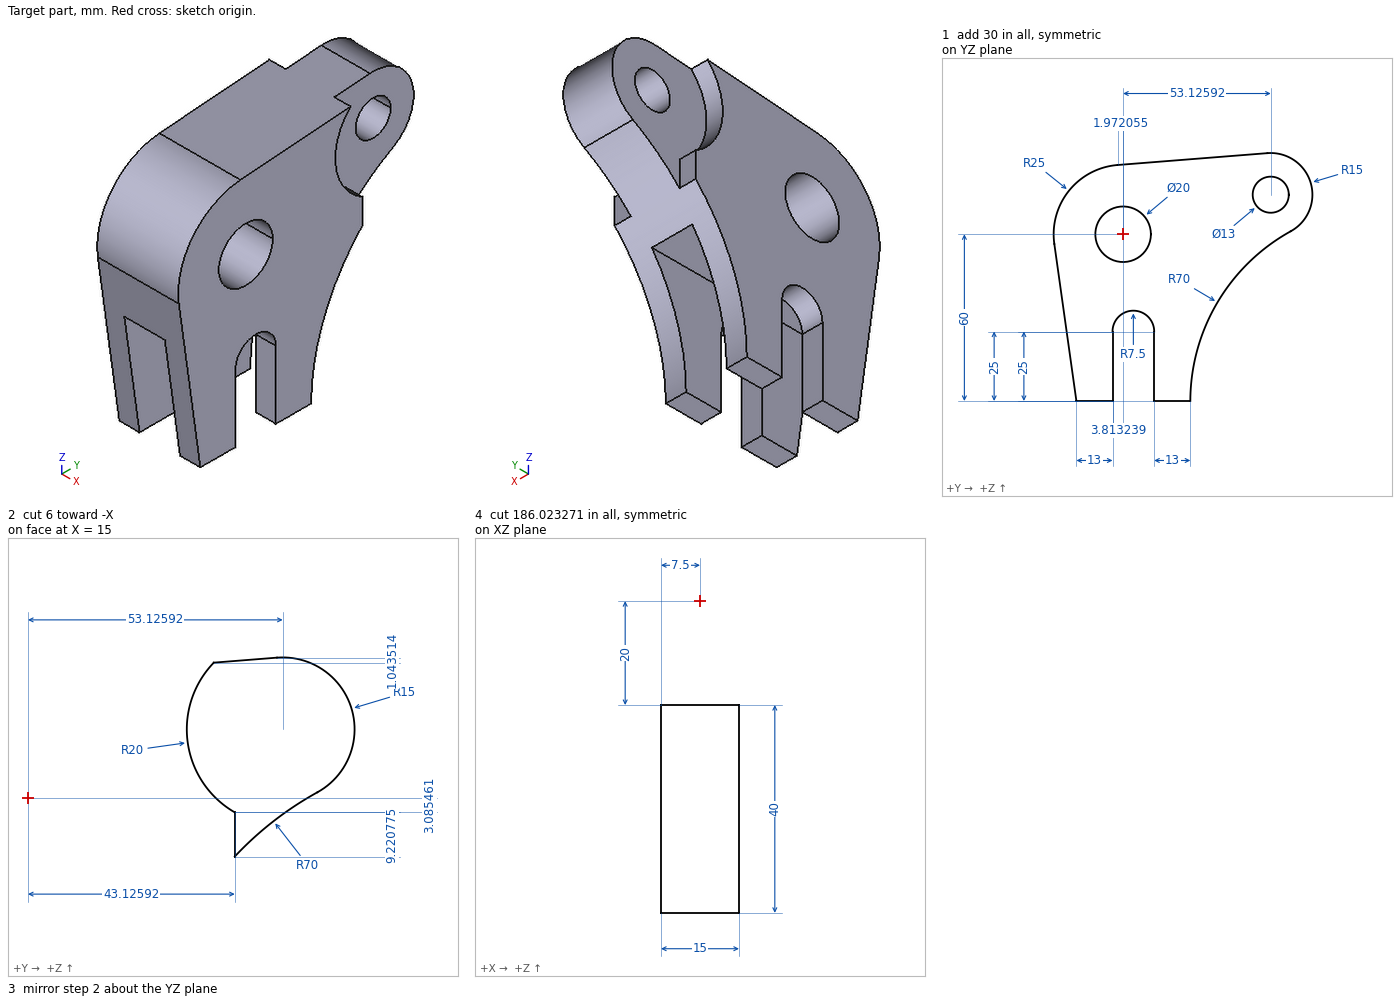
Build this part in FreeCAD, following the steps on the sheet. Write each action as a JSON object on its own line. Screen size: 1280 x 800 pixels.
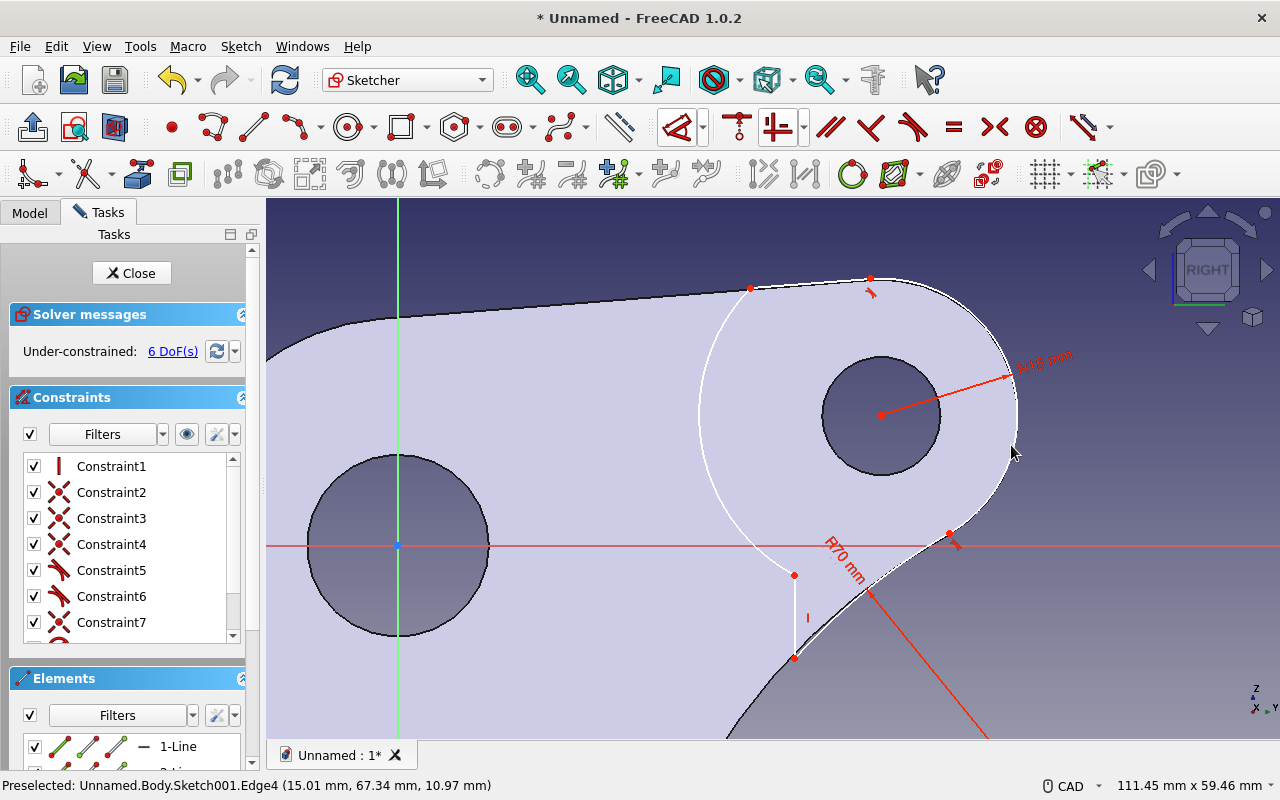
{"action": "left_click", "coordinate": [703, 376]}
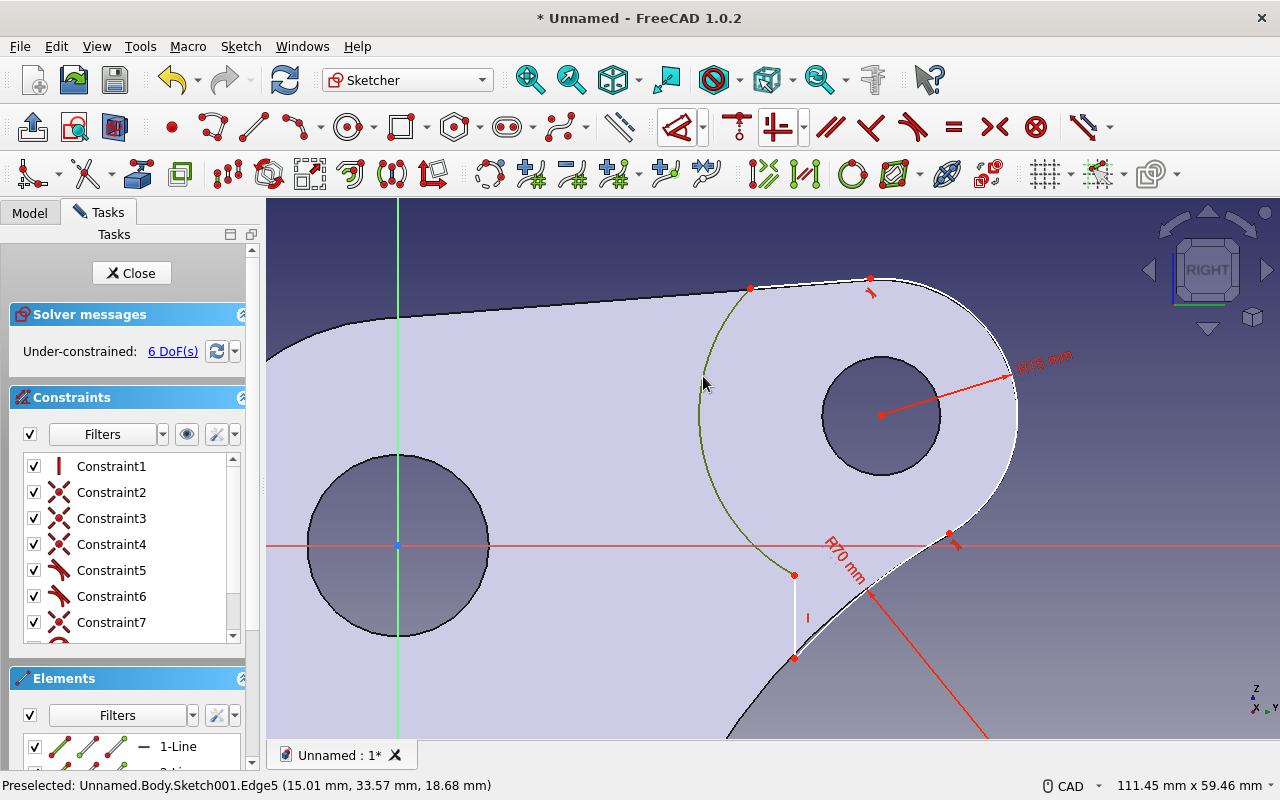
{"action": "left_click", "coordinate": [702, 128]}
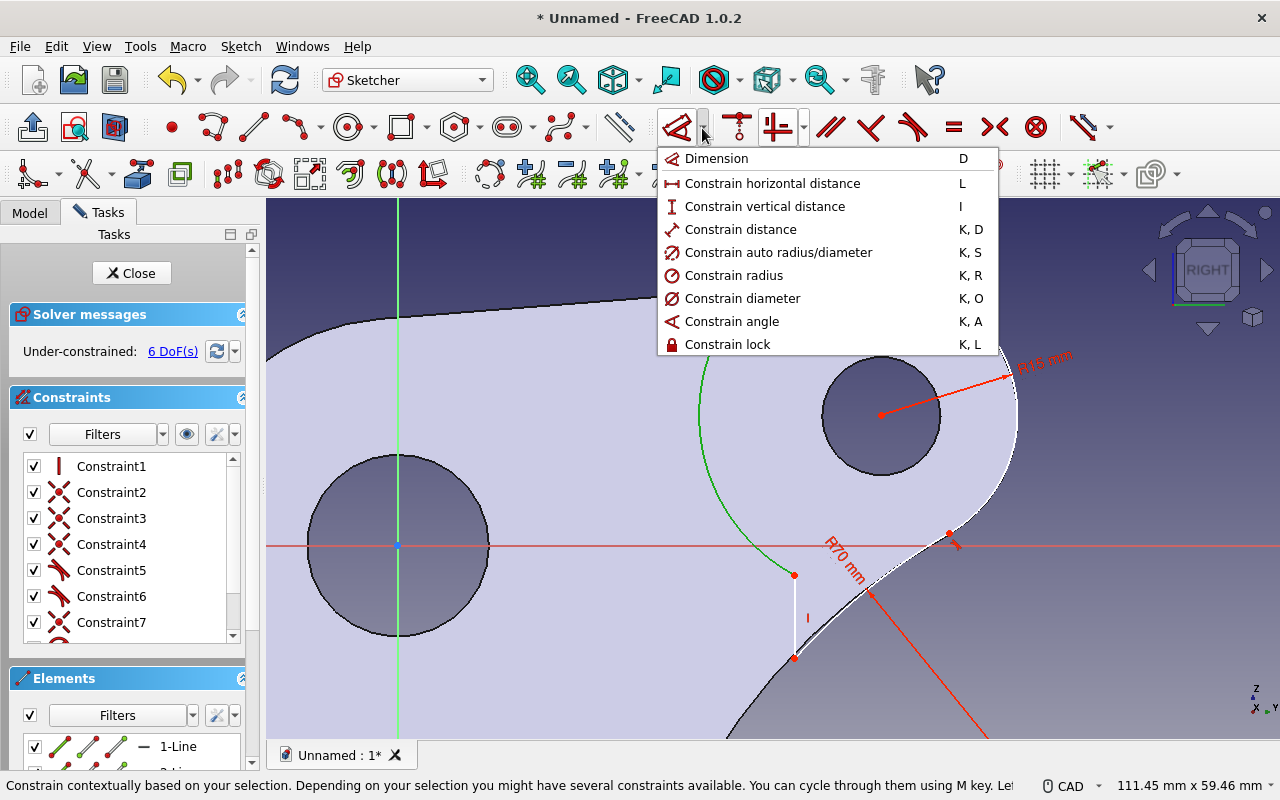
{"action": "left_click", "coordinate": [828, 276]}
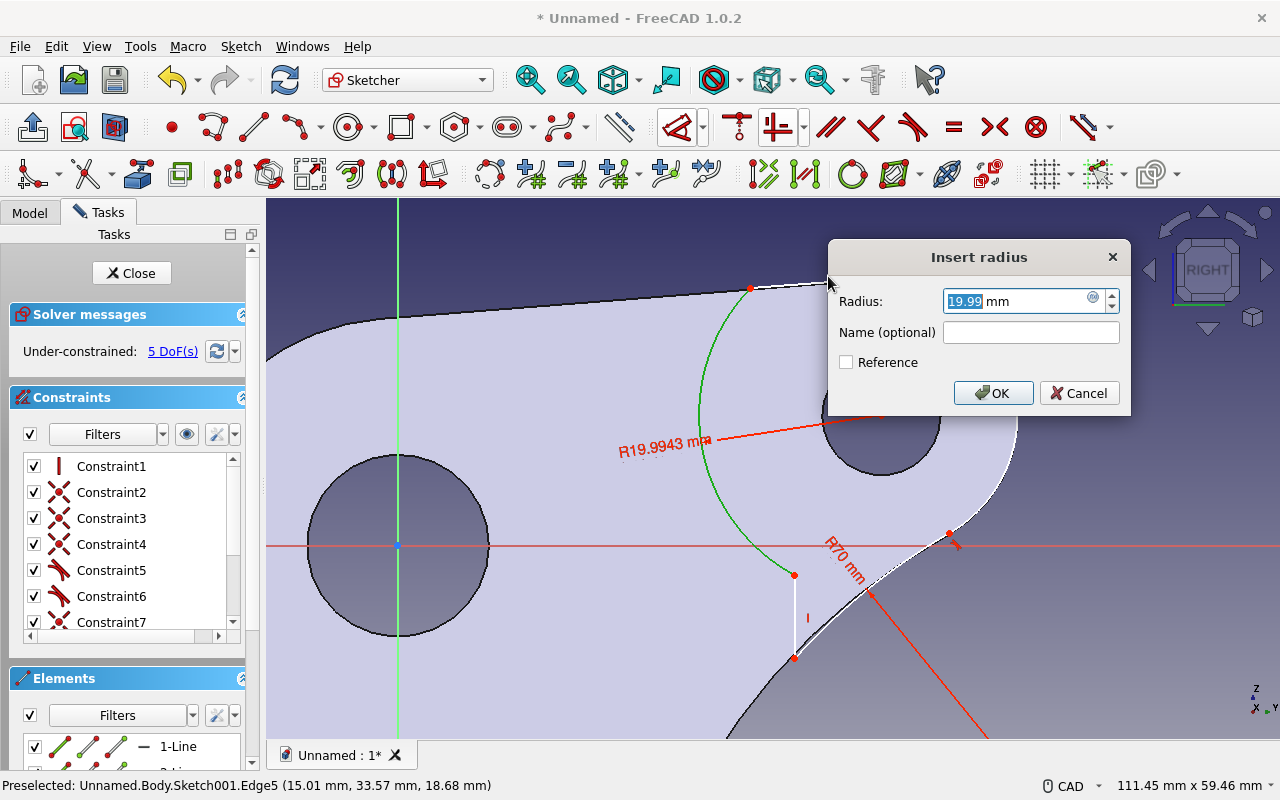
{"action": "type", "text": "20"}
{"action": "key", "text": "Return"}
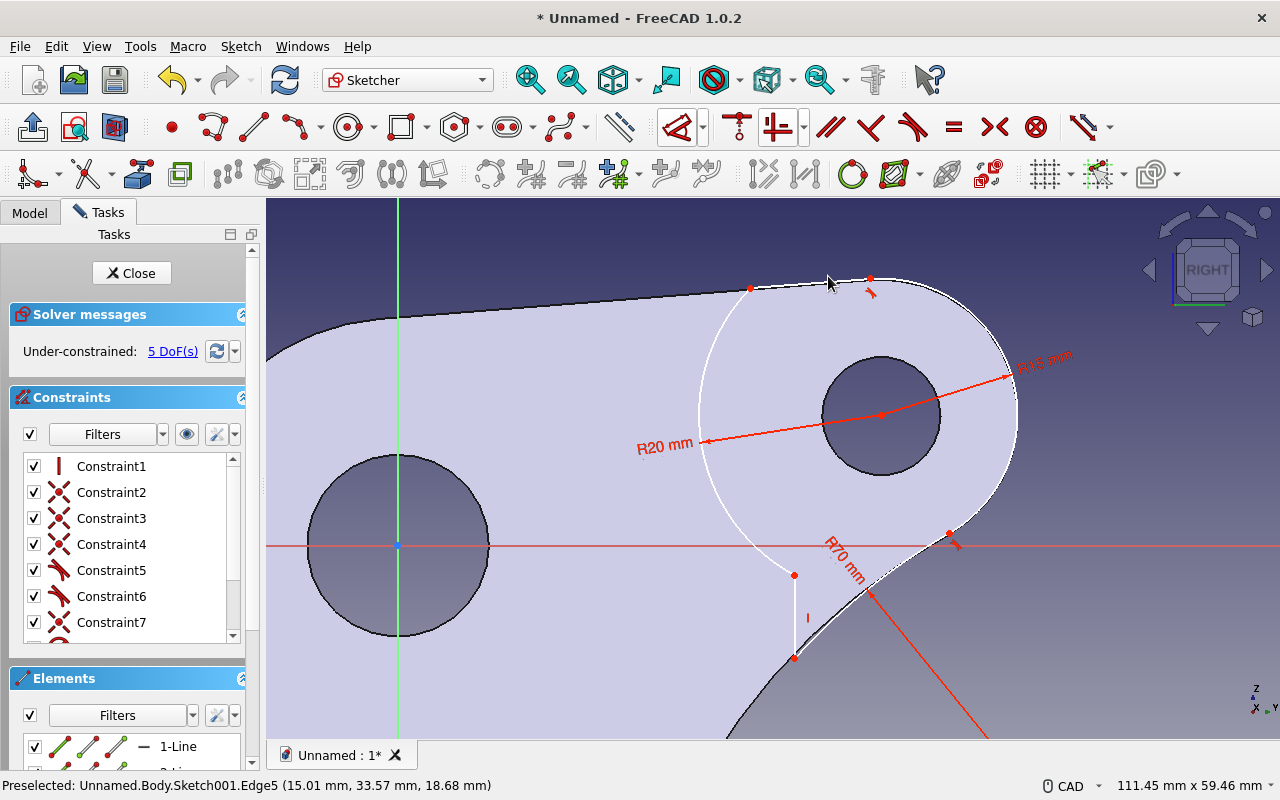
{"action": "left_click", "coordinate": [795, 600]}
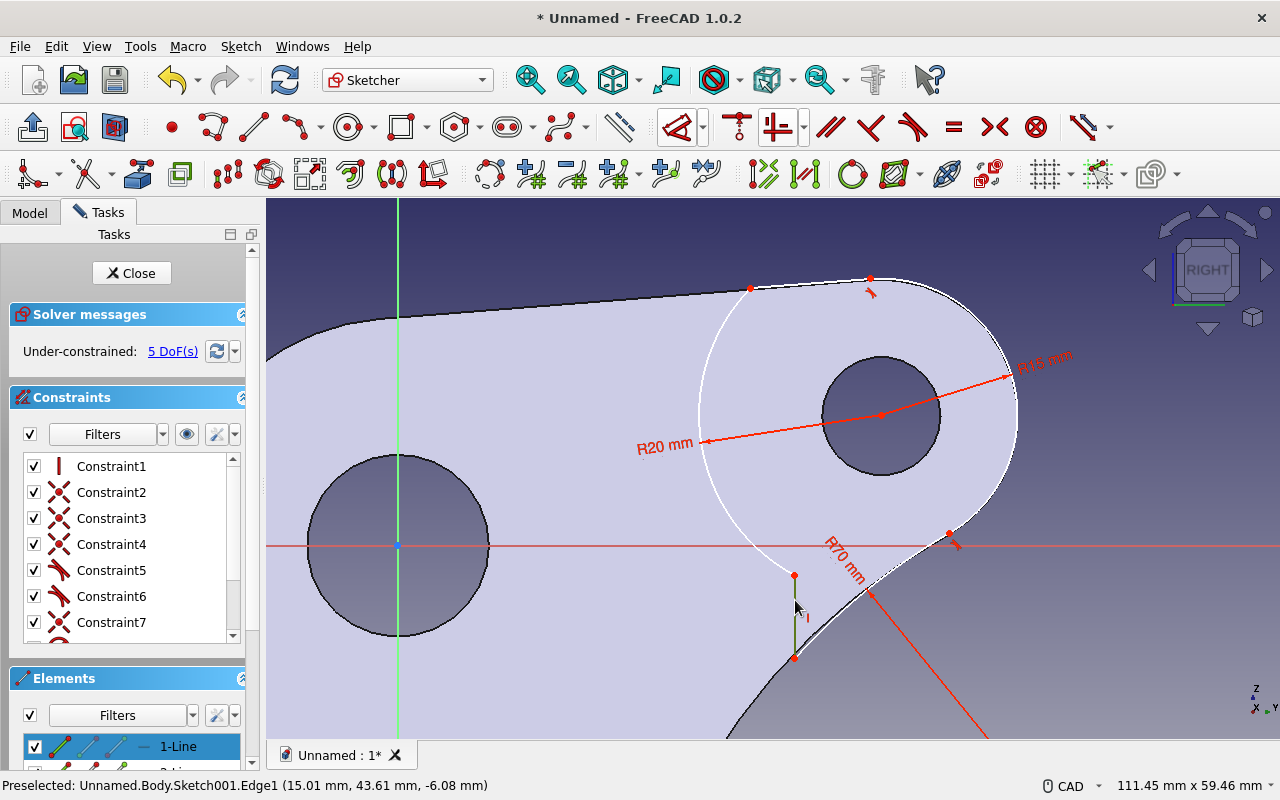
{"action": "left_click", "coordinate": [702, 128]}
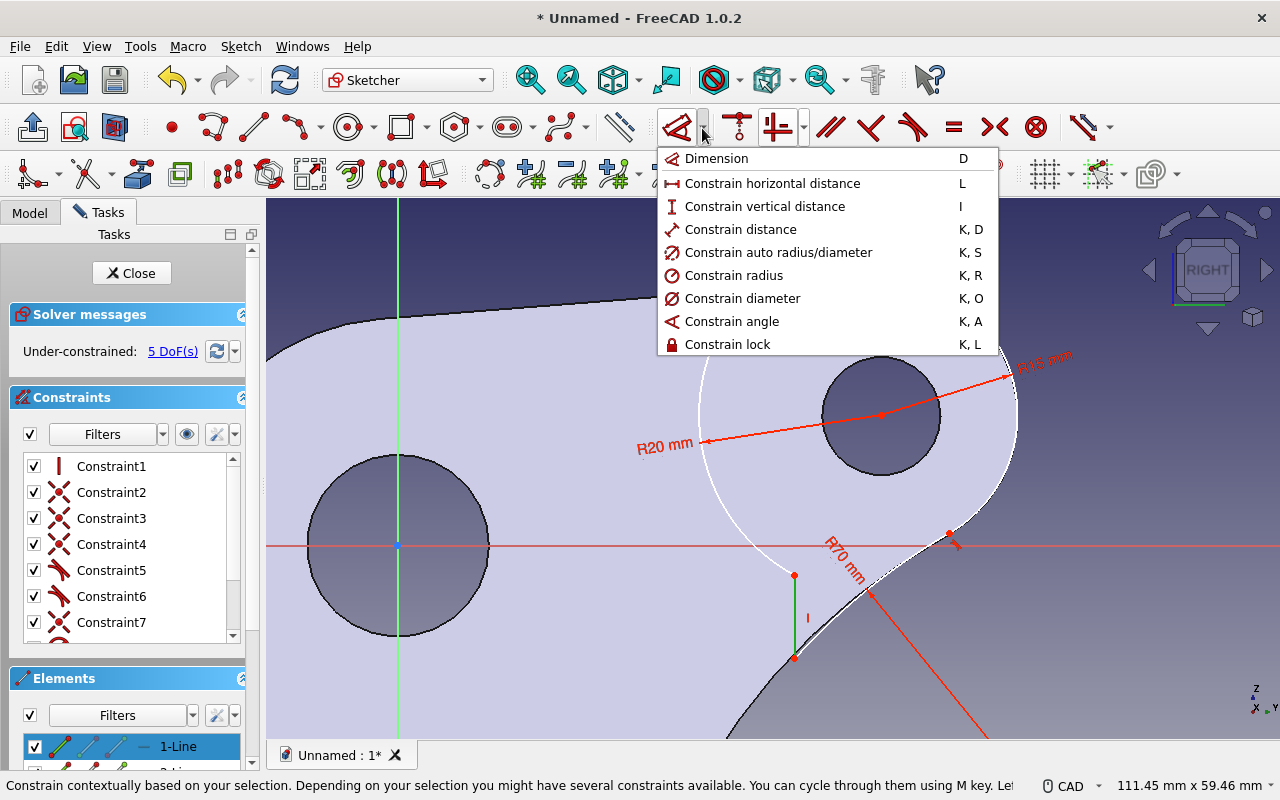
{"action": "left_click", "coordinate": [828, 206]}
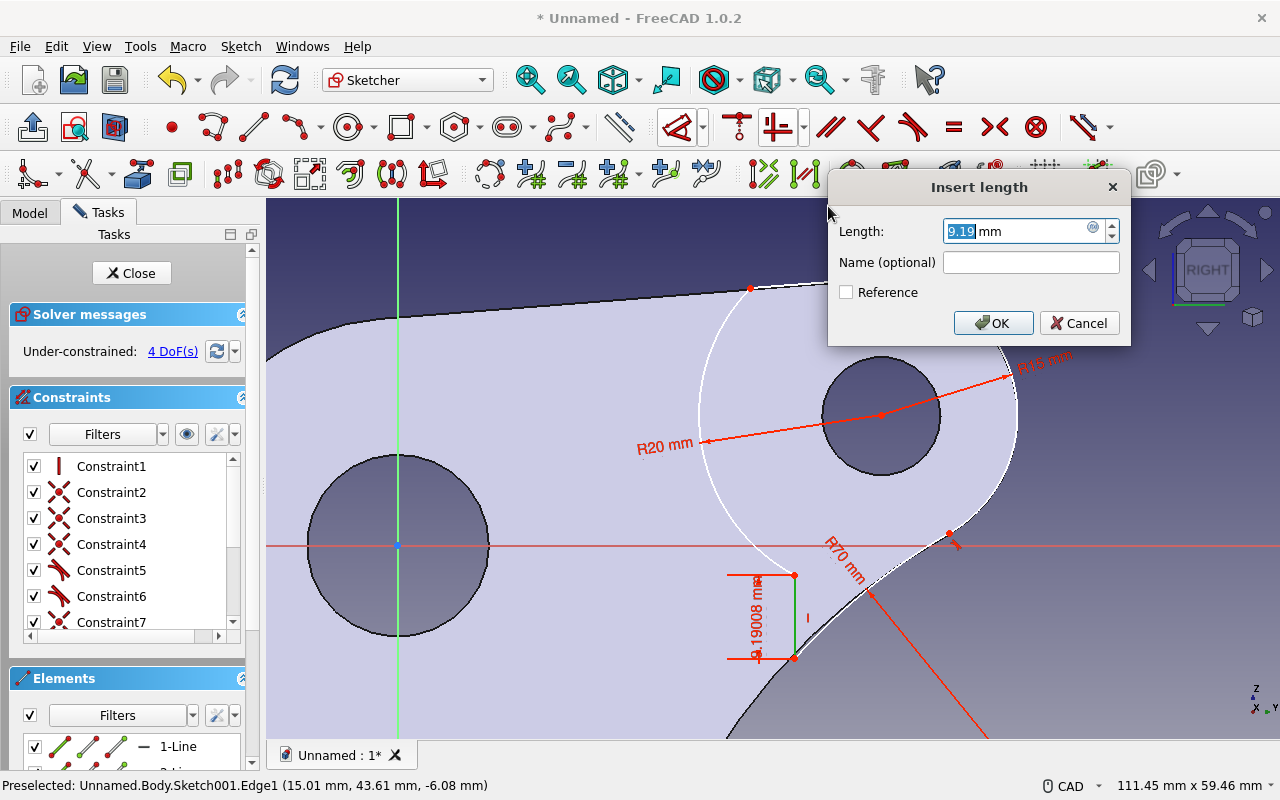
{"action": "type", "text": "9.220775"}
{"action": "key", "text": "Return"}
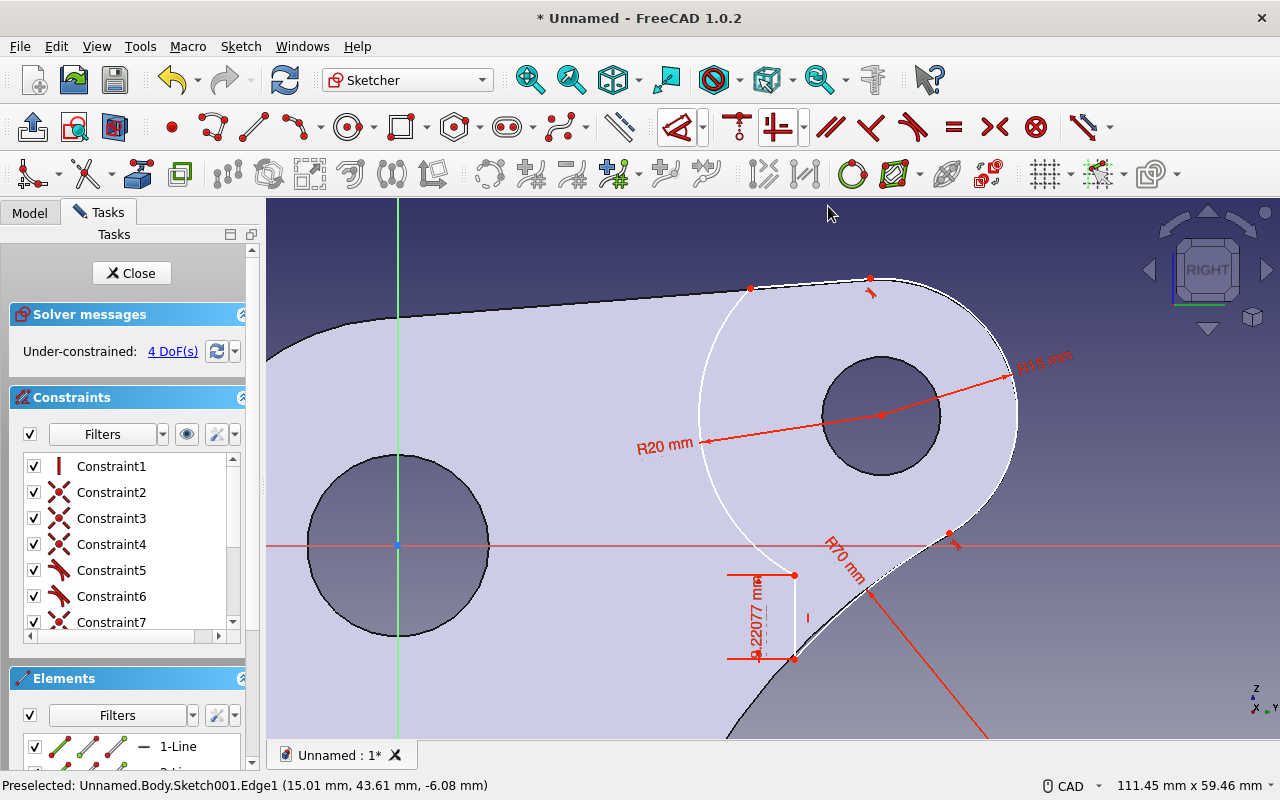
{"action": "left_click", "coordinate": [795, 575]}